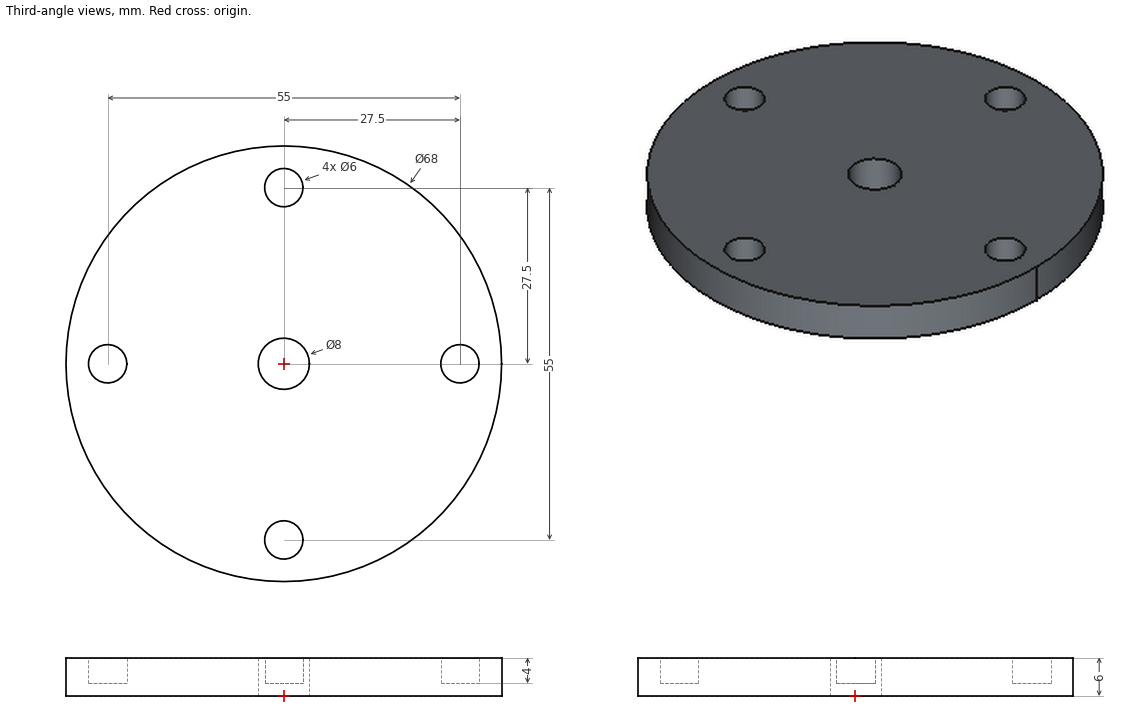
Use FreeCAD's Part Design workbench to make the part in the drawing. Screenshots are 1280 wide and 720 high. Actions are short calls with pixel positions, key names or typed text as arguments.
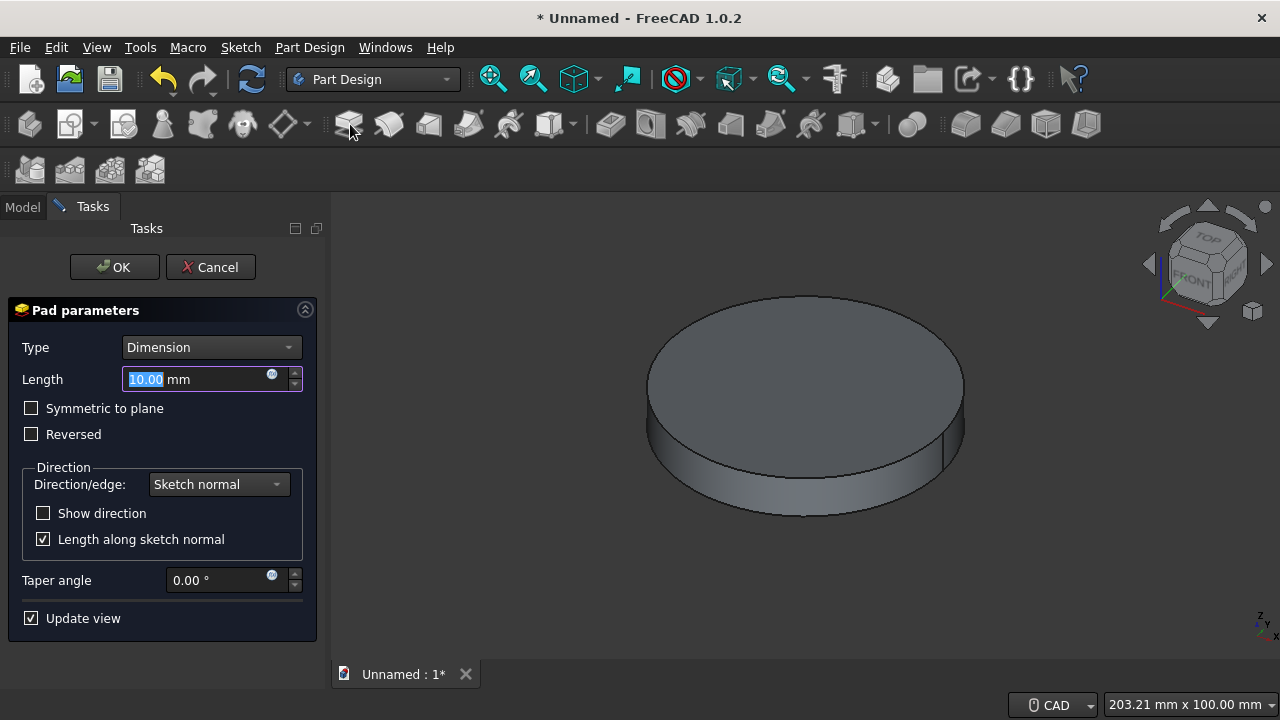
text(6)
key(Tab)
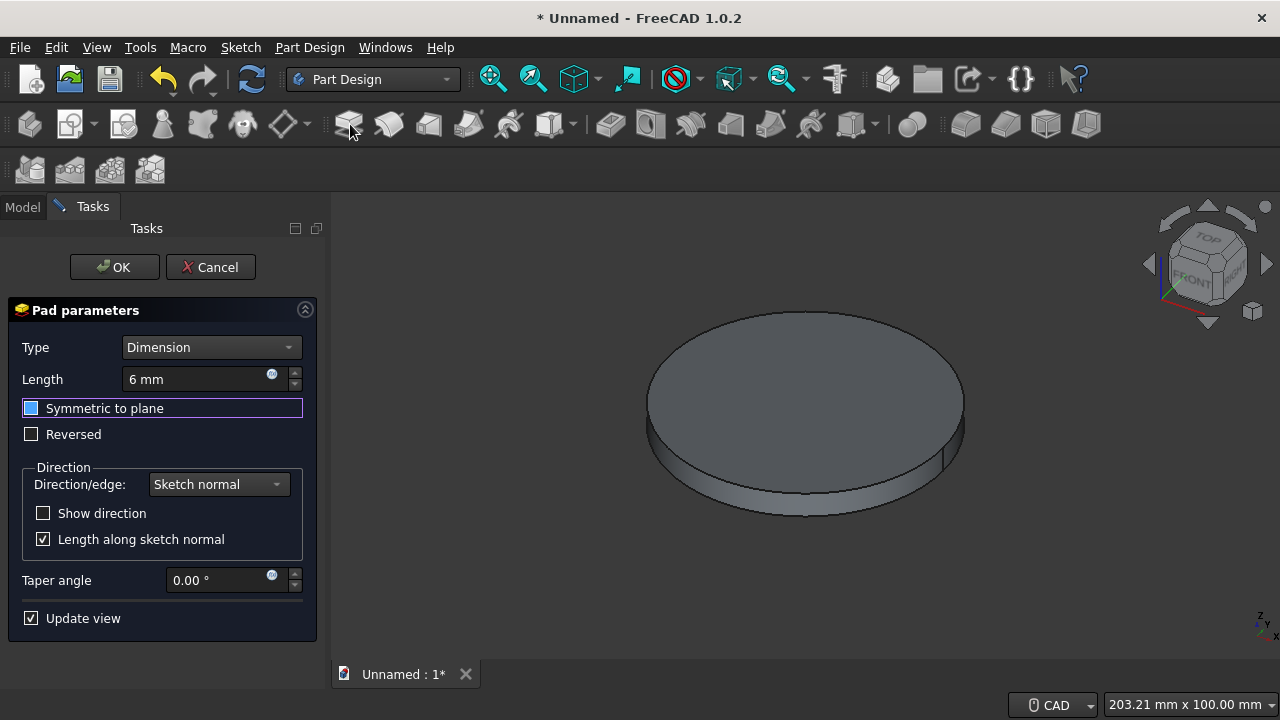
click(115, 267)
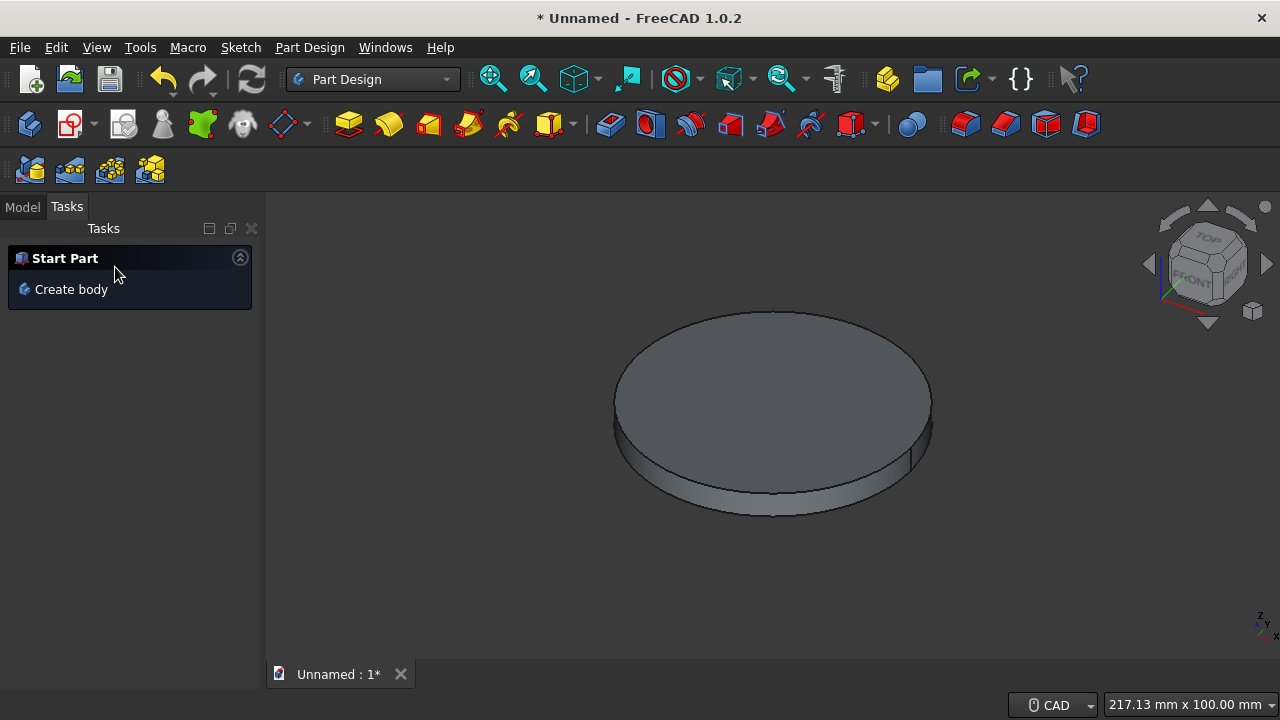
click(773, 402)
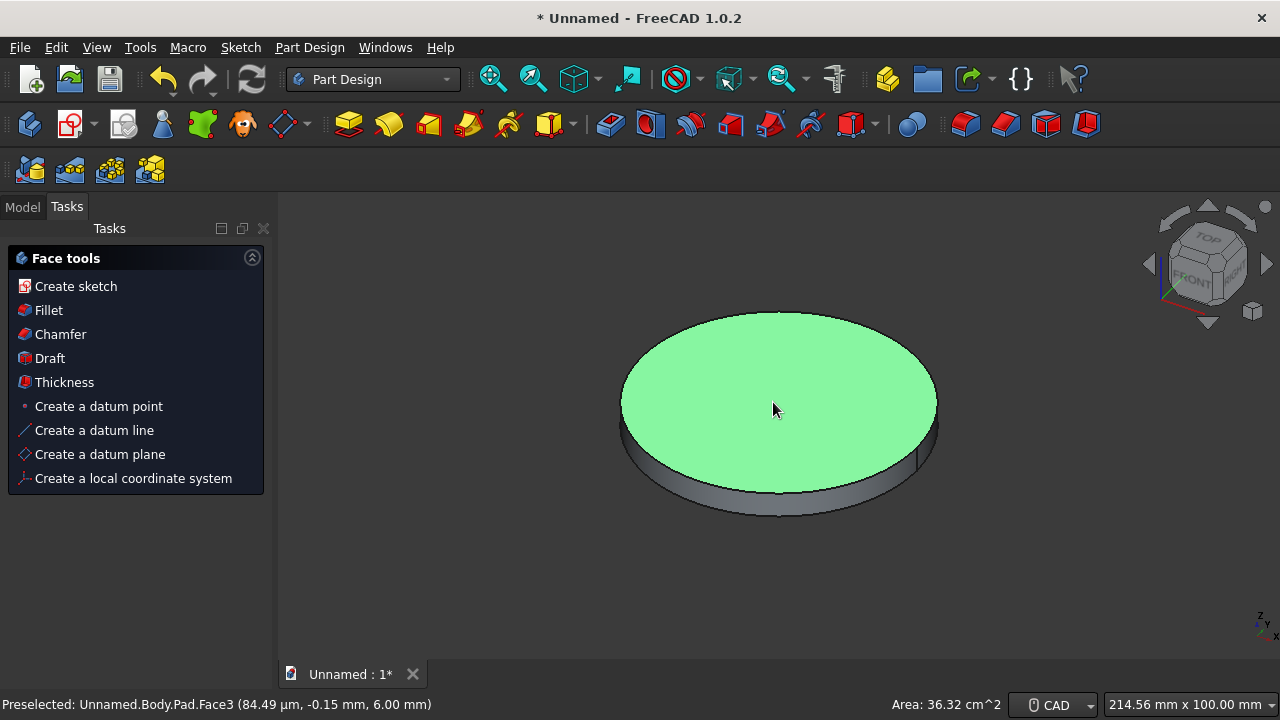
click(70, 124)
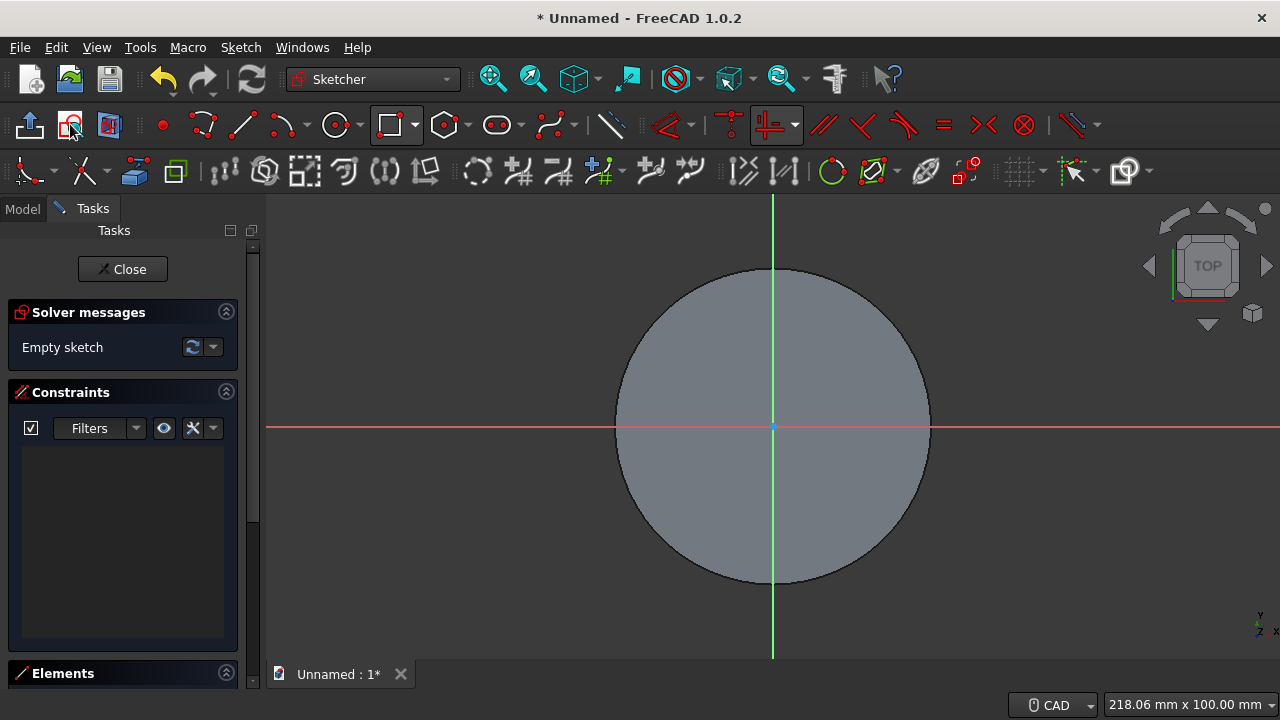
key(g)
key(c)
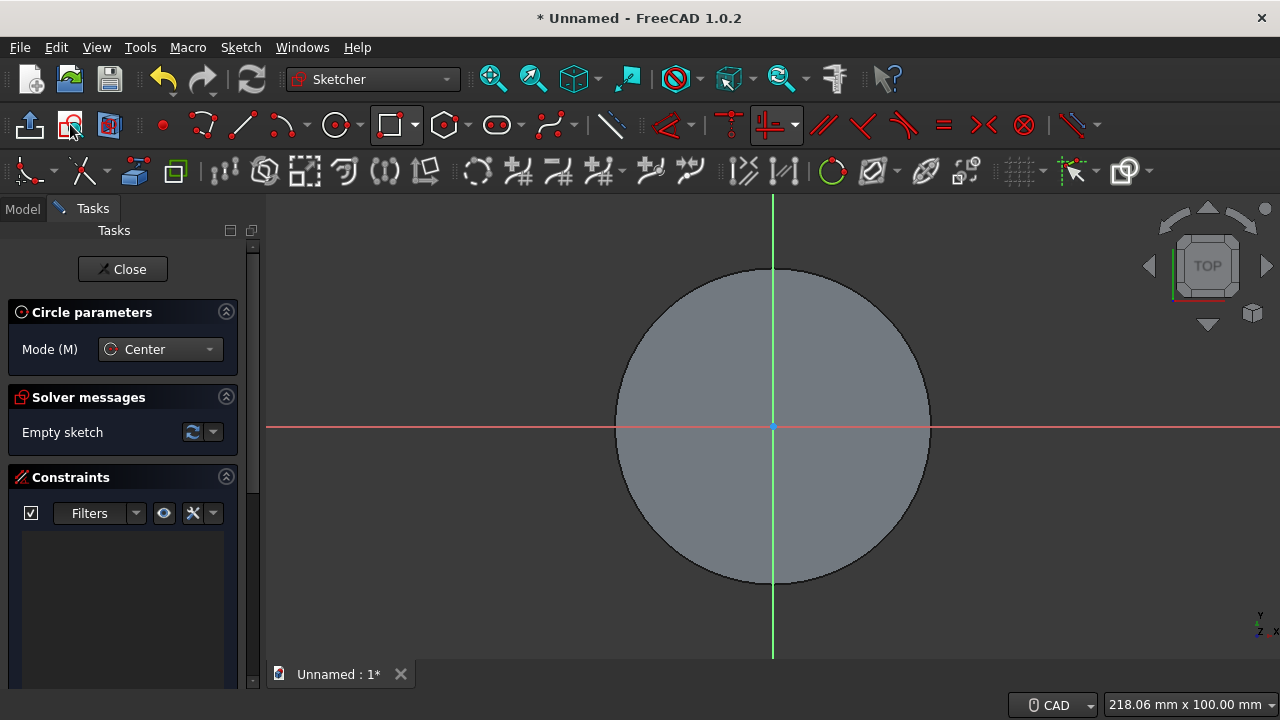
scroll(773, 299, up, 3)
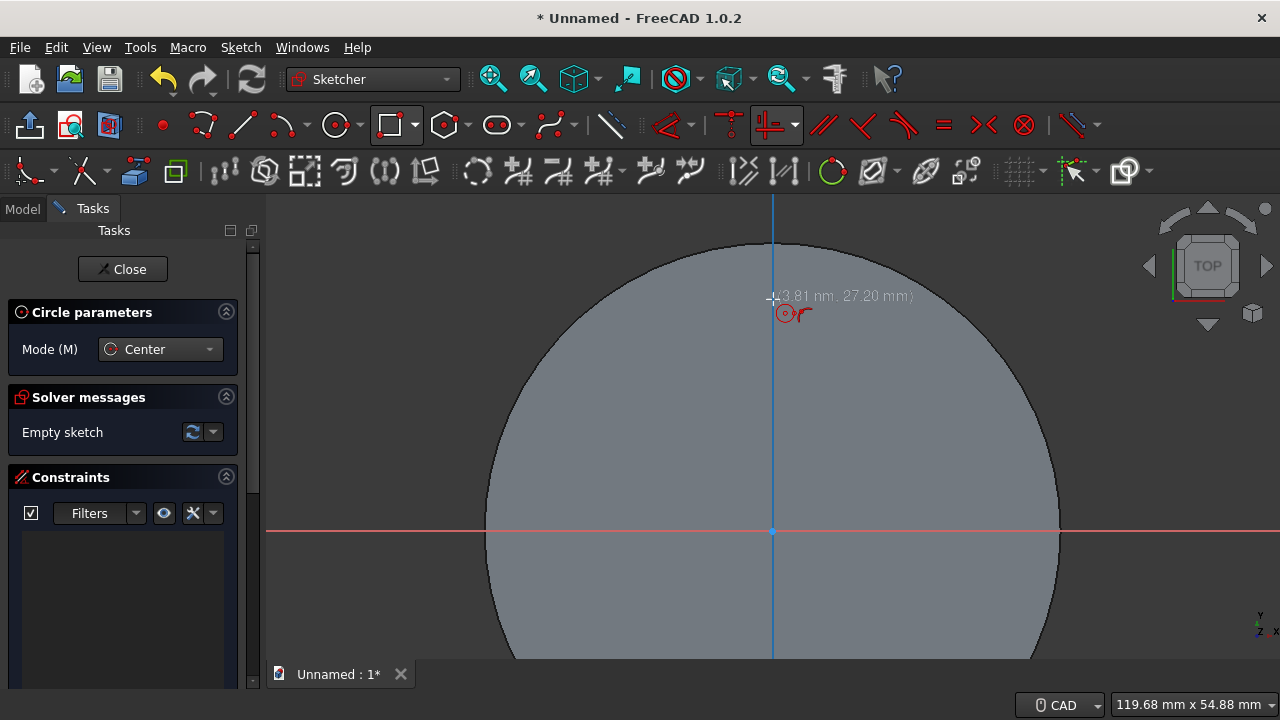
click(773, 298)
click(791, 280)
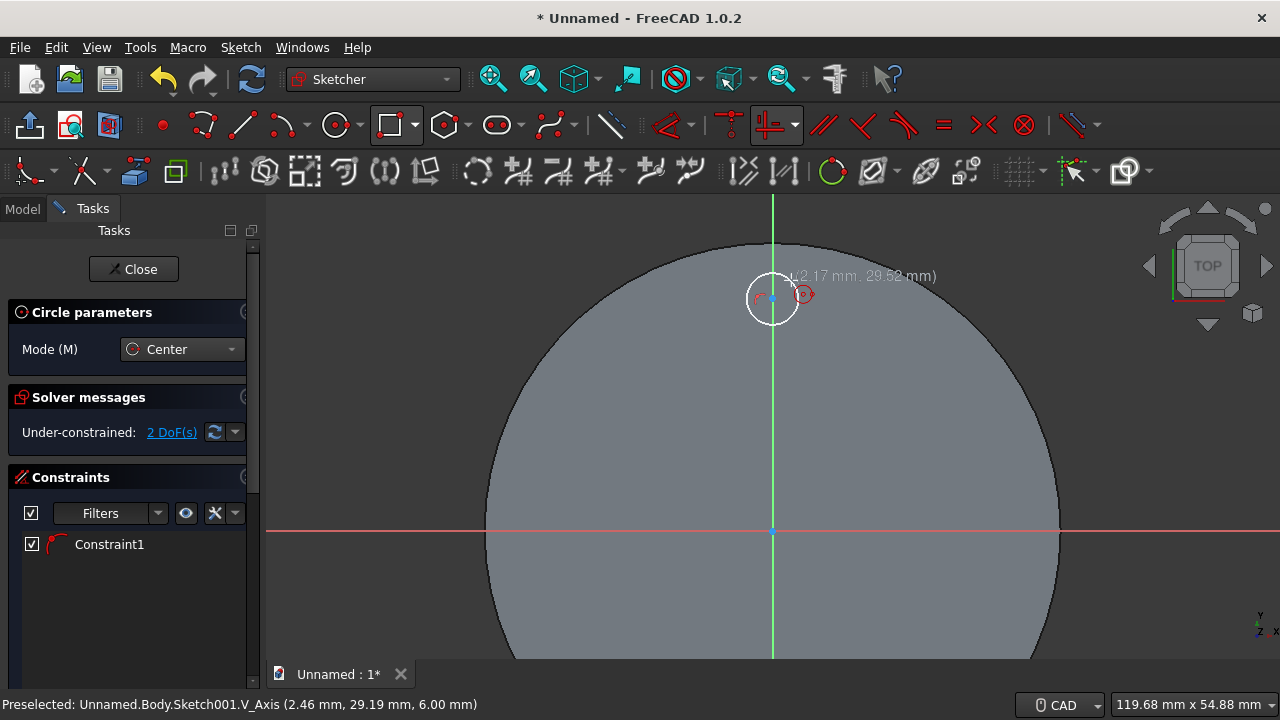
click(1006, 531)
click(1024, 513)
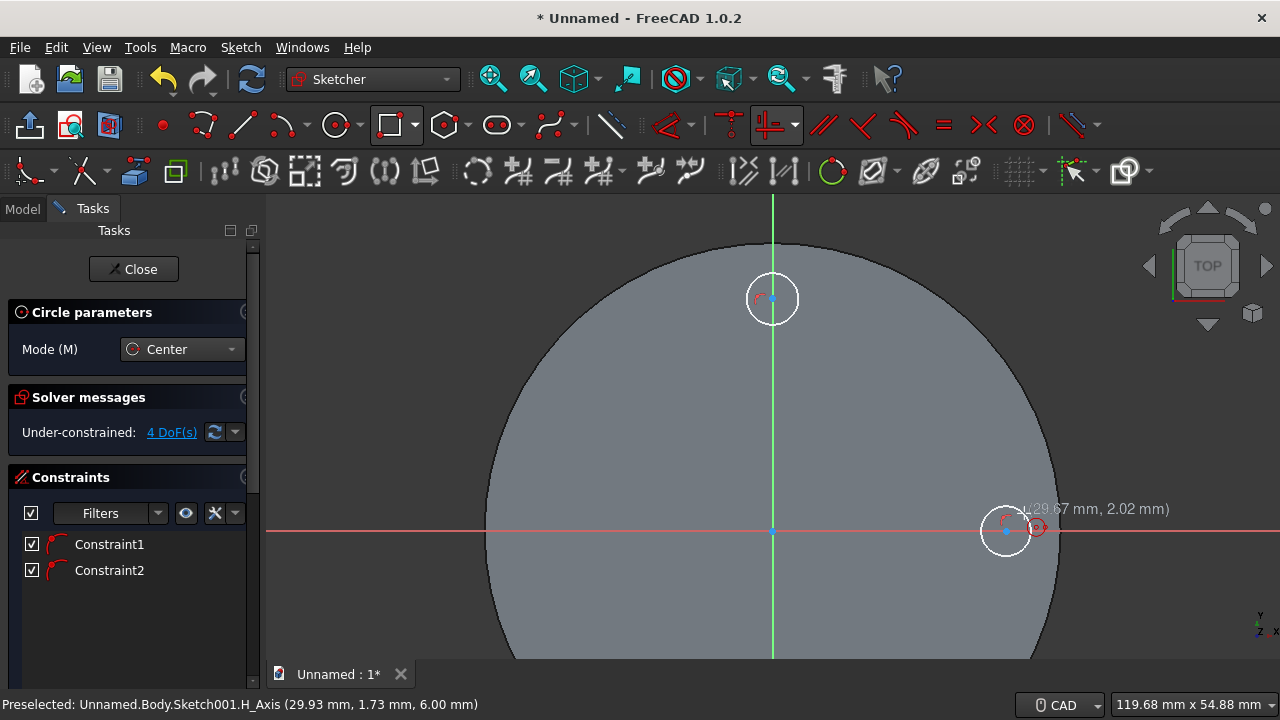
scroll(622, 299, down, 3)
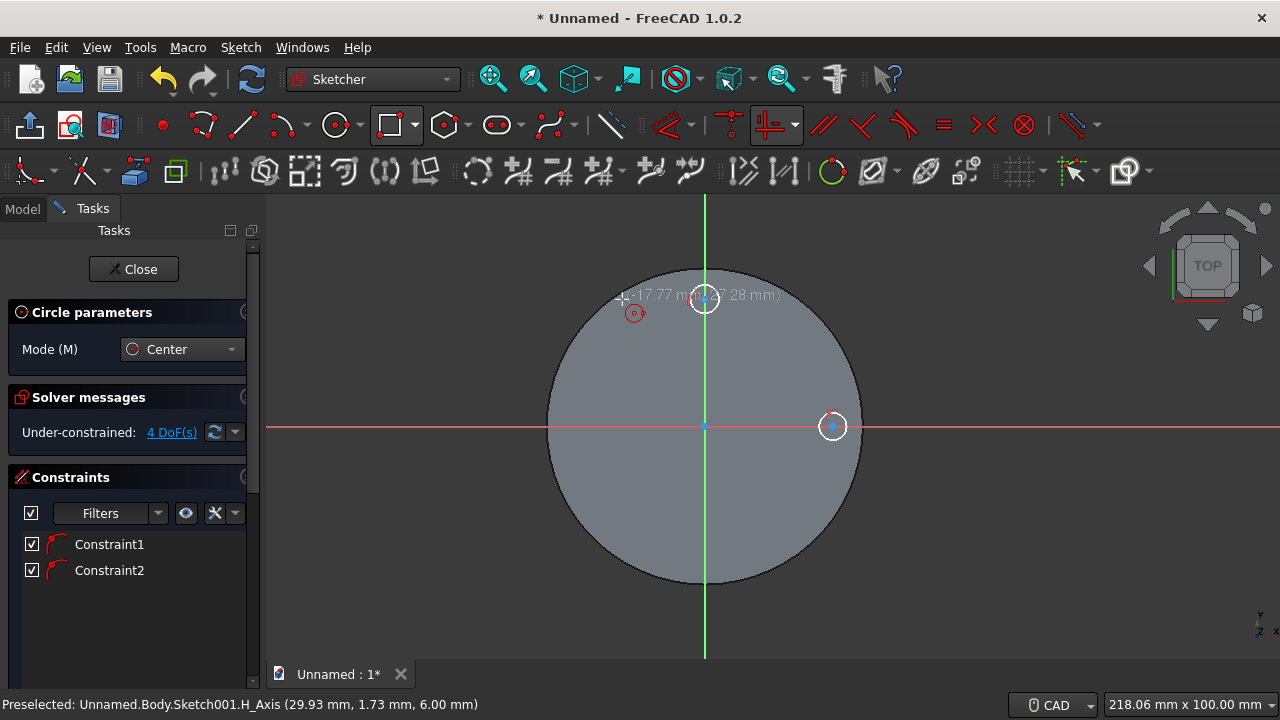
scroll(705, 554, up, 3)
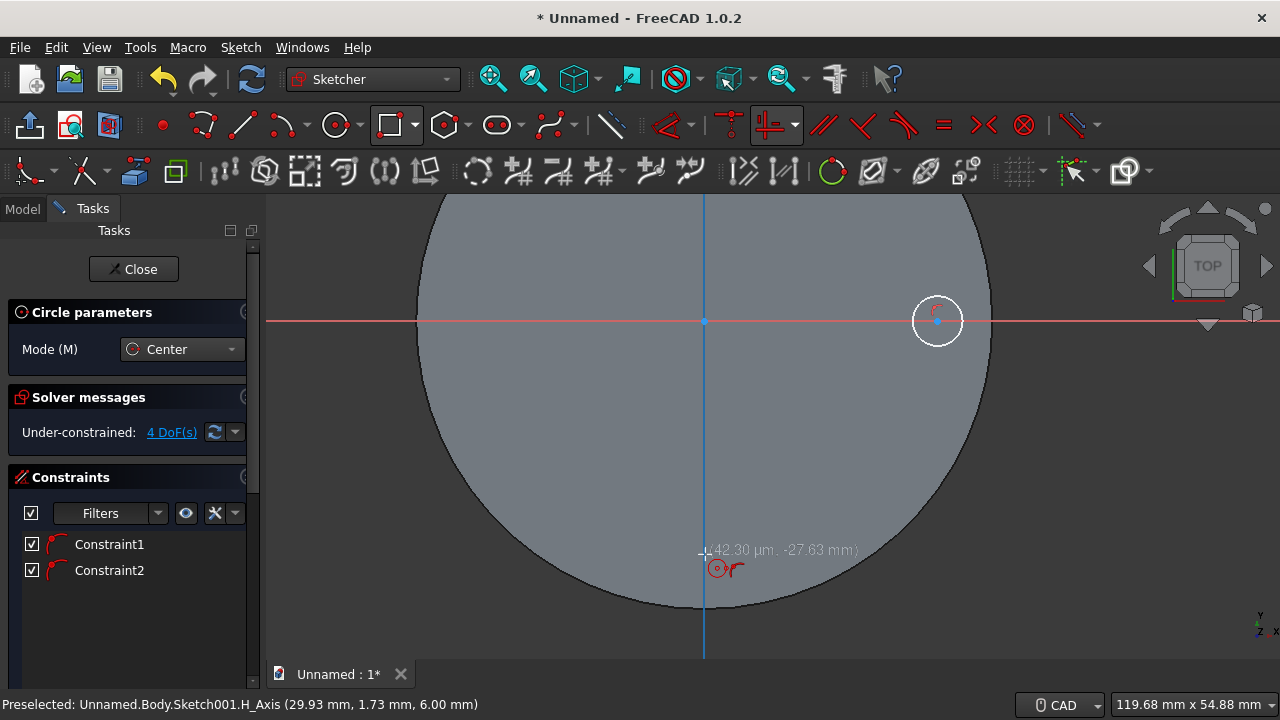
click(704, 554)
click(722, 536)